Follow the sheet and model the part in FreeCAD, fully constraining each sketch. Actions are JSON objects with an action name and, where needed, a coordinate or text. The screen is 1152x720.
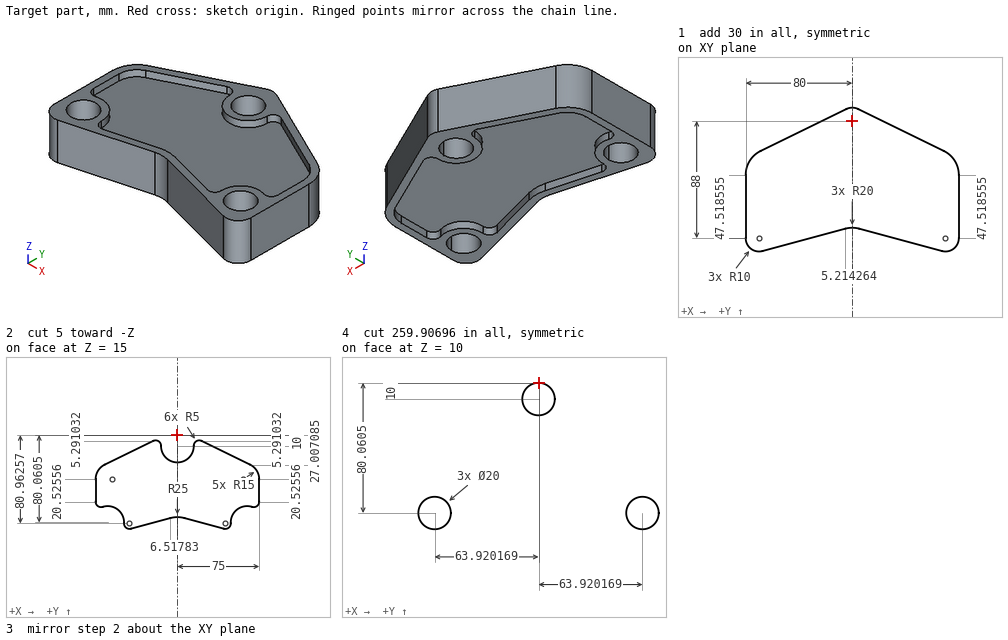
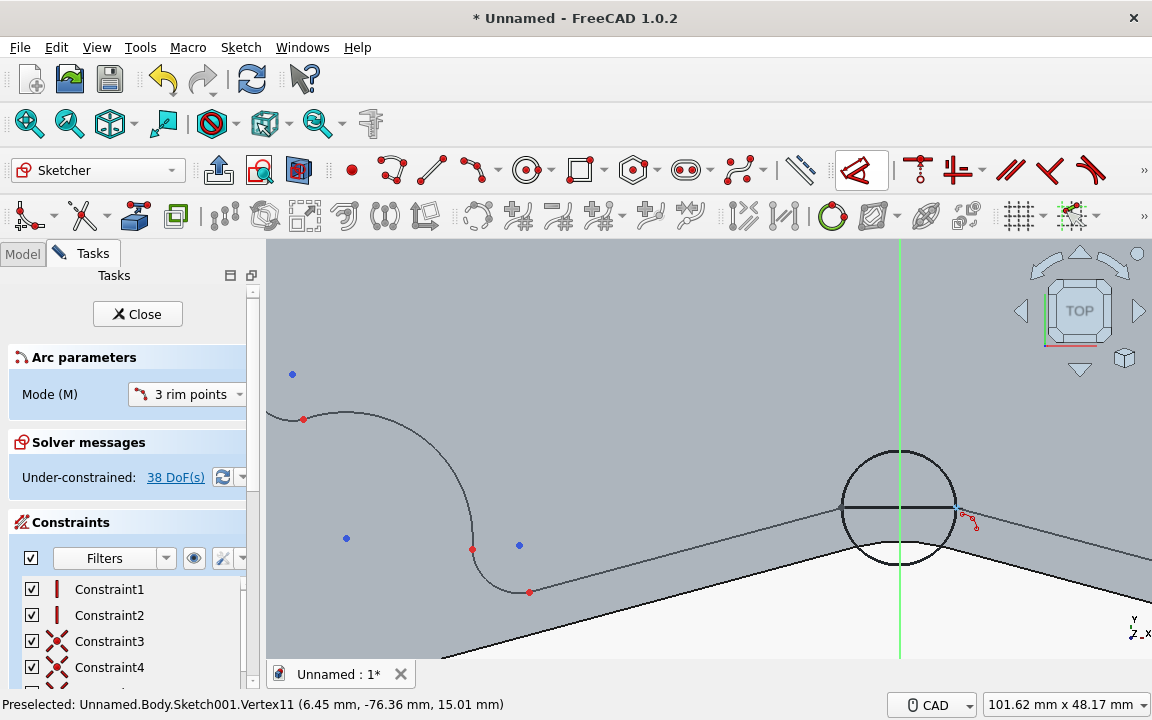
{"action": "scroll", "coordinate": [911, 498], "scroll_direction": "up", "scroll_amount": 4}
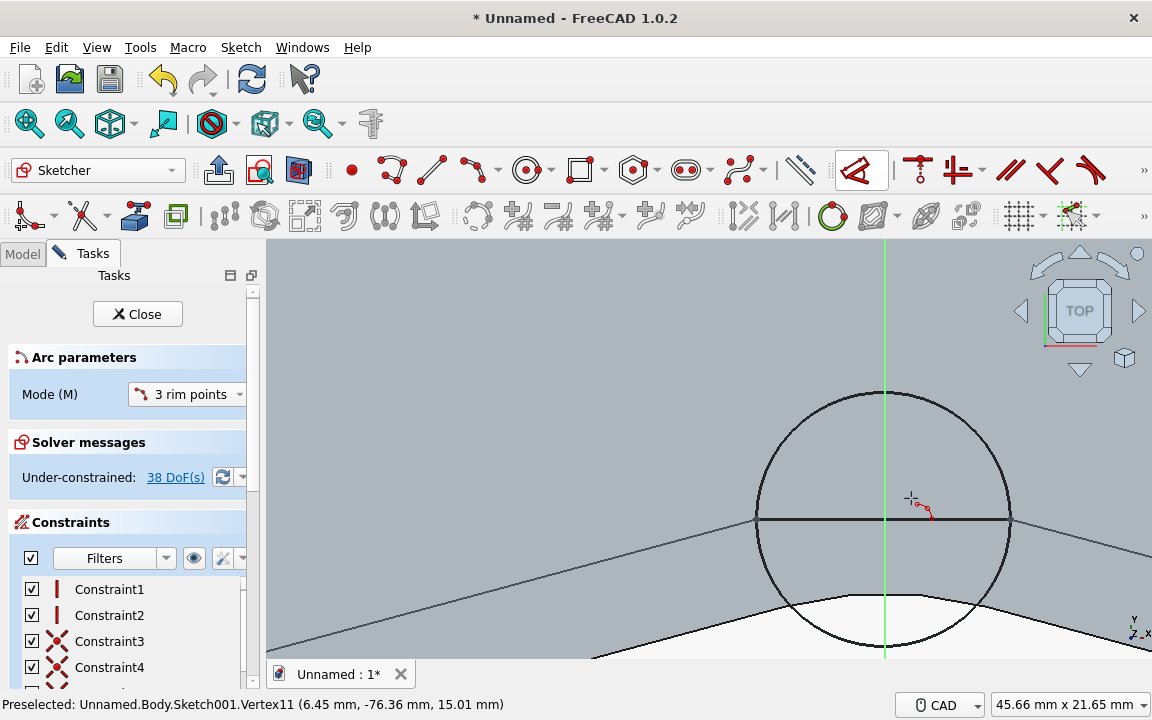
{"action": "left_click", "coordinate": [911, 497]}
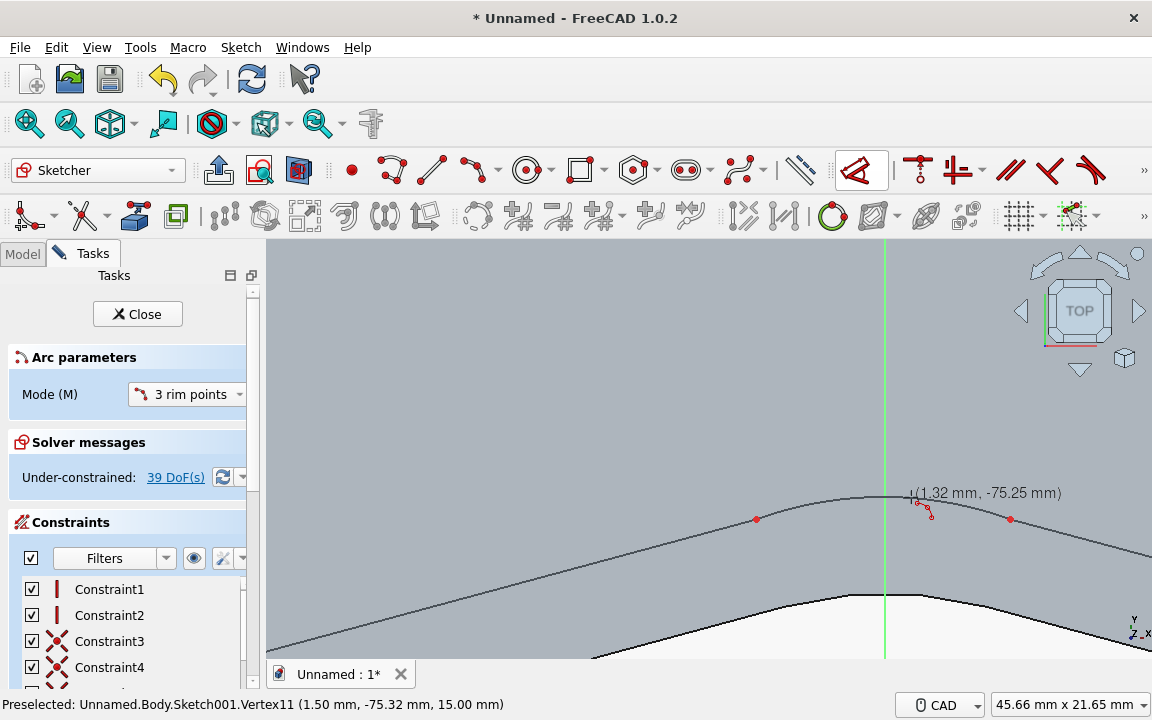
{"action": "scroll", "coordinate": [592, 564], "scroll_direction": "down", "scroll_amount": 9}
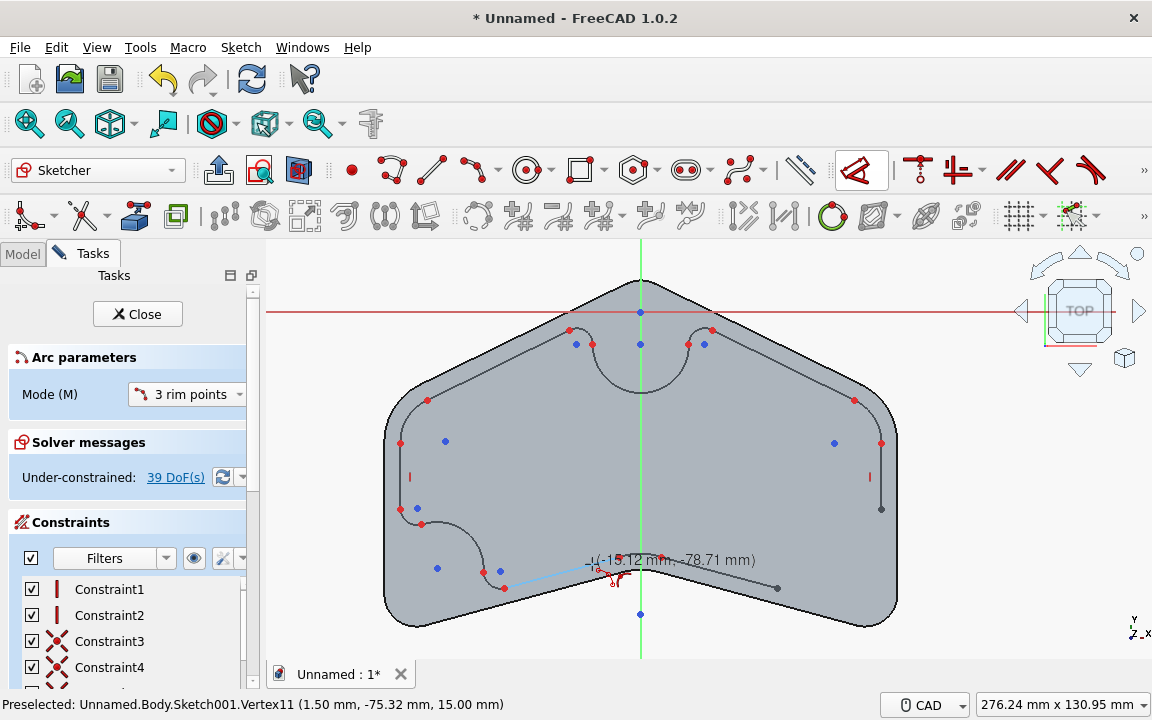
{"action": "left_click", "coordinate": [777, 588]}
{"action": "left_click", "coordinate": [798, 571]}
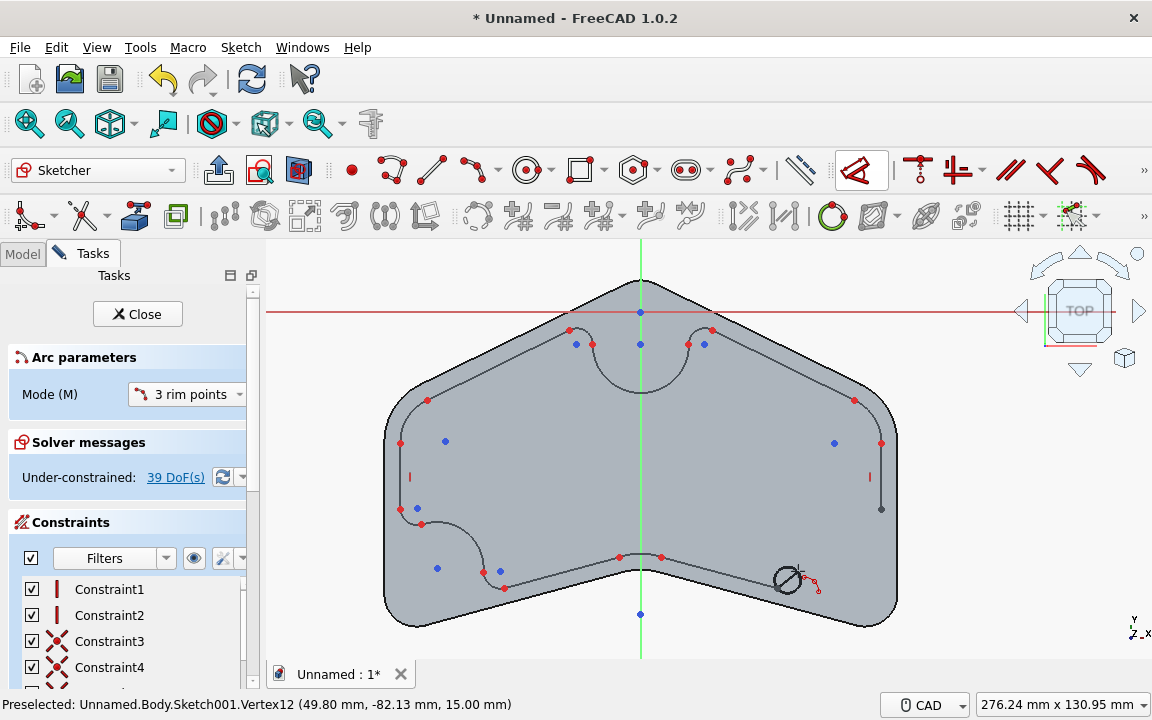
{"action": "scroll", "coordinate": [792, 585], "scroll_direction": "up", "scroll_amount": 5}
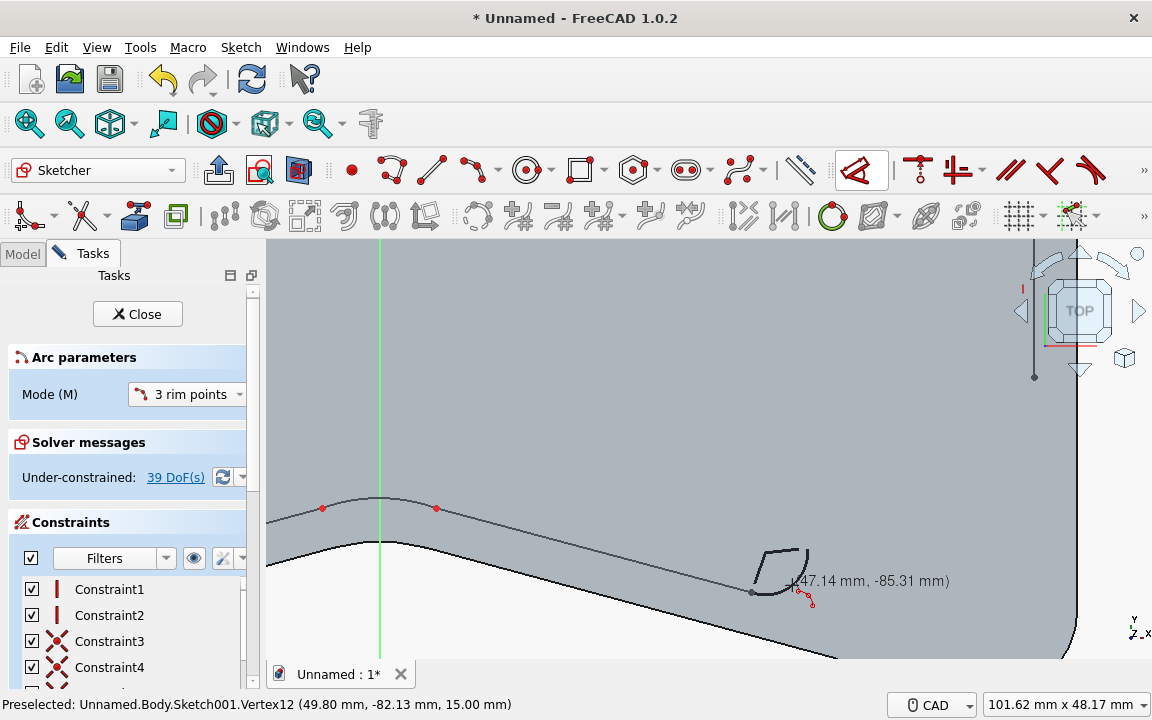
{"action": "left_click", "coordinate": [790, 582]}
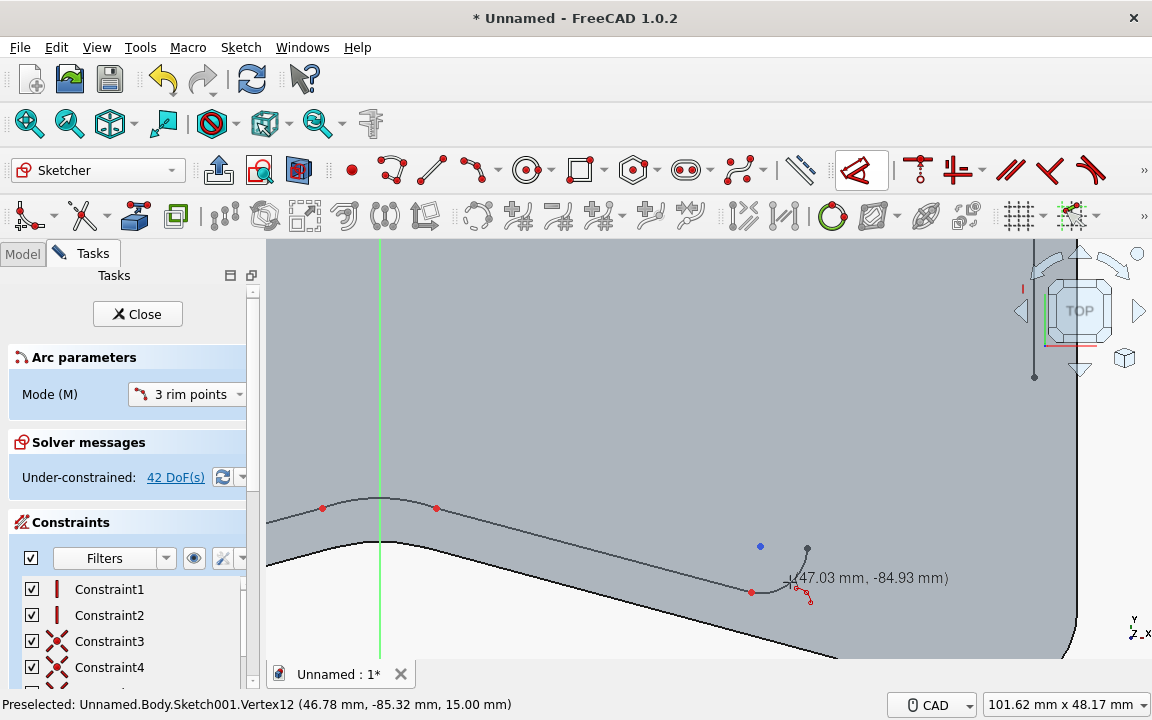
{"action": "left_click", "coordinate": [807, 548]}
{"action": "left_click", "coordinate": [977, 416]}
{"action": "left_click", "coordinate": [858, 437]}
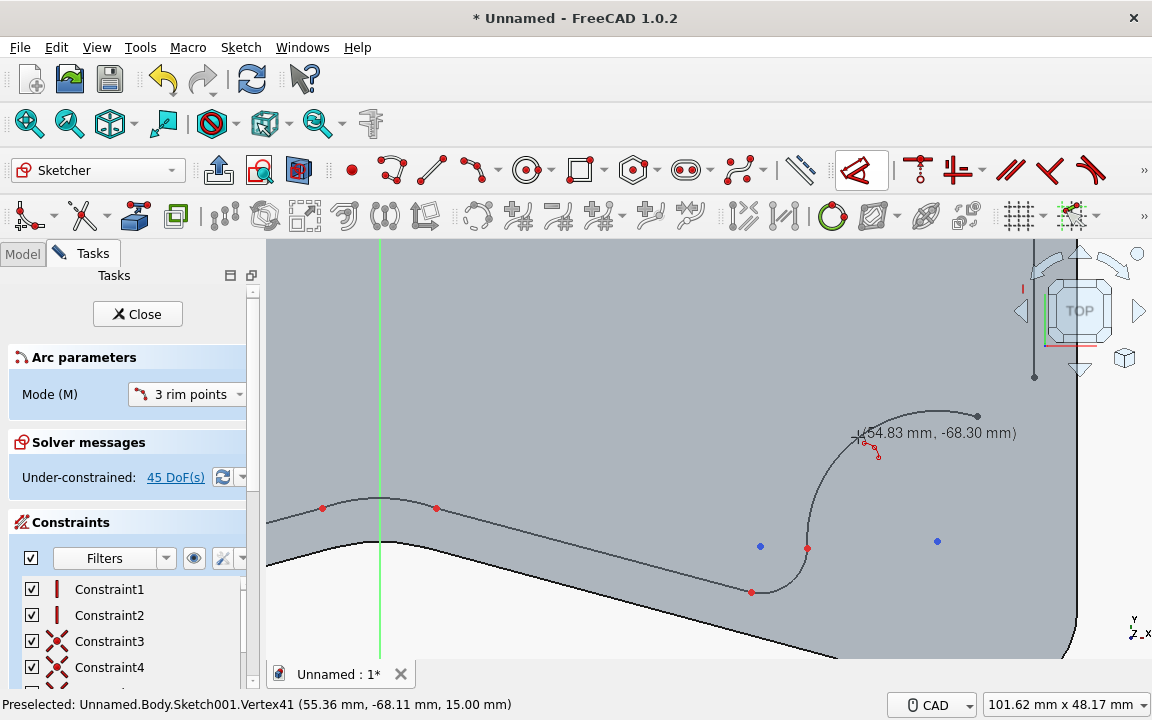
{"action": "left_click", "coordinate": [977, 417]}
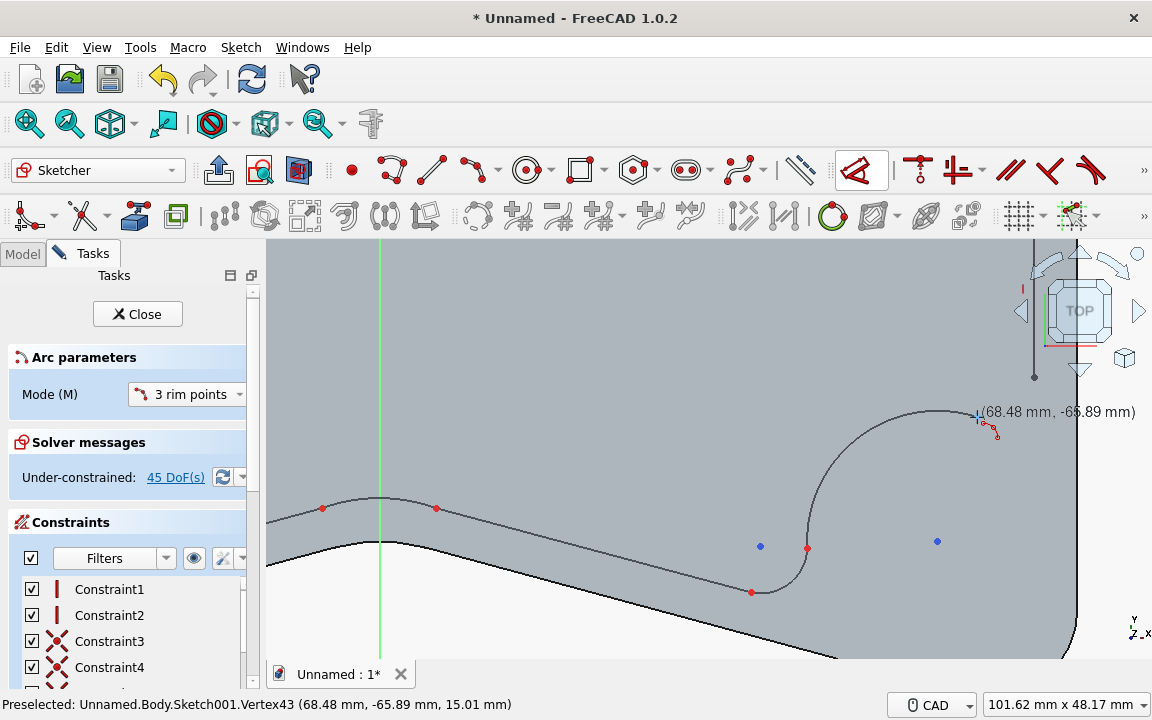
{"action": "scroll", "coordinate": [792, 584], "scroll_direction": "down", "scroll_amount": 5}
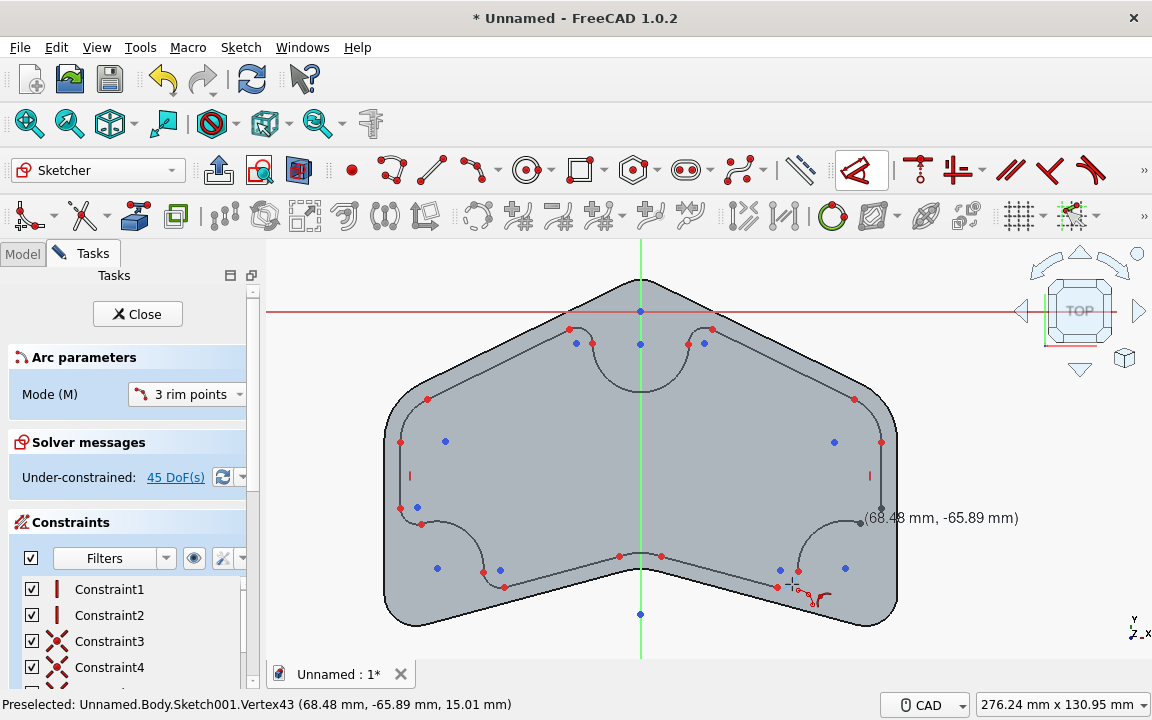
{"action": "left_click", "coordinate": [881, 509]}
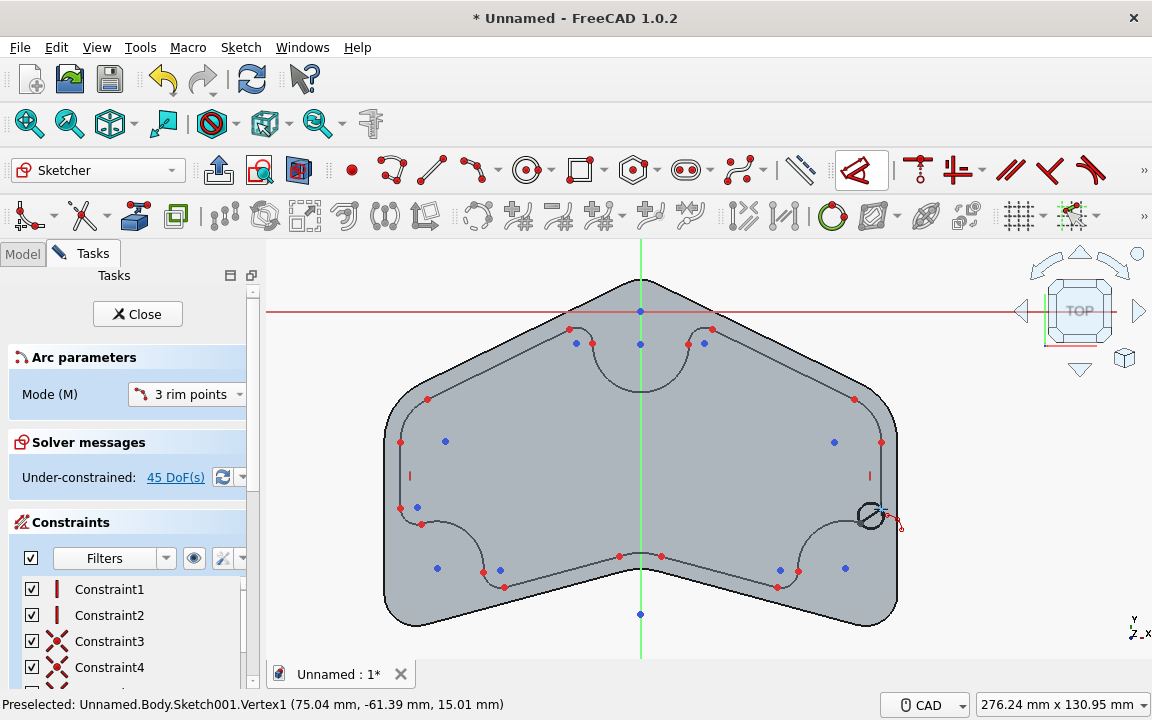
{"action": "scroll", "coordinate": [875, 520], "scroll_direction": "up", "scroll_amount": 5}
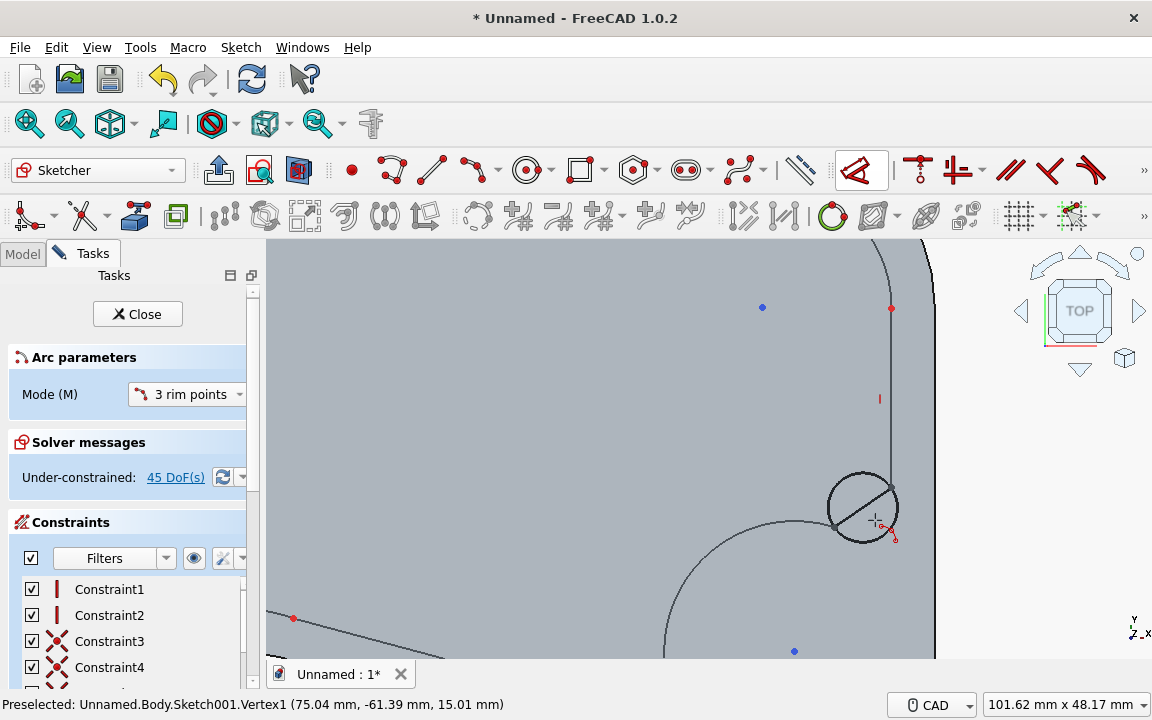
{"action": "left_click", "coordinate": [873, 520]}
{"action": "key", "text": "Escape"}